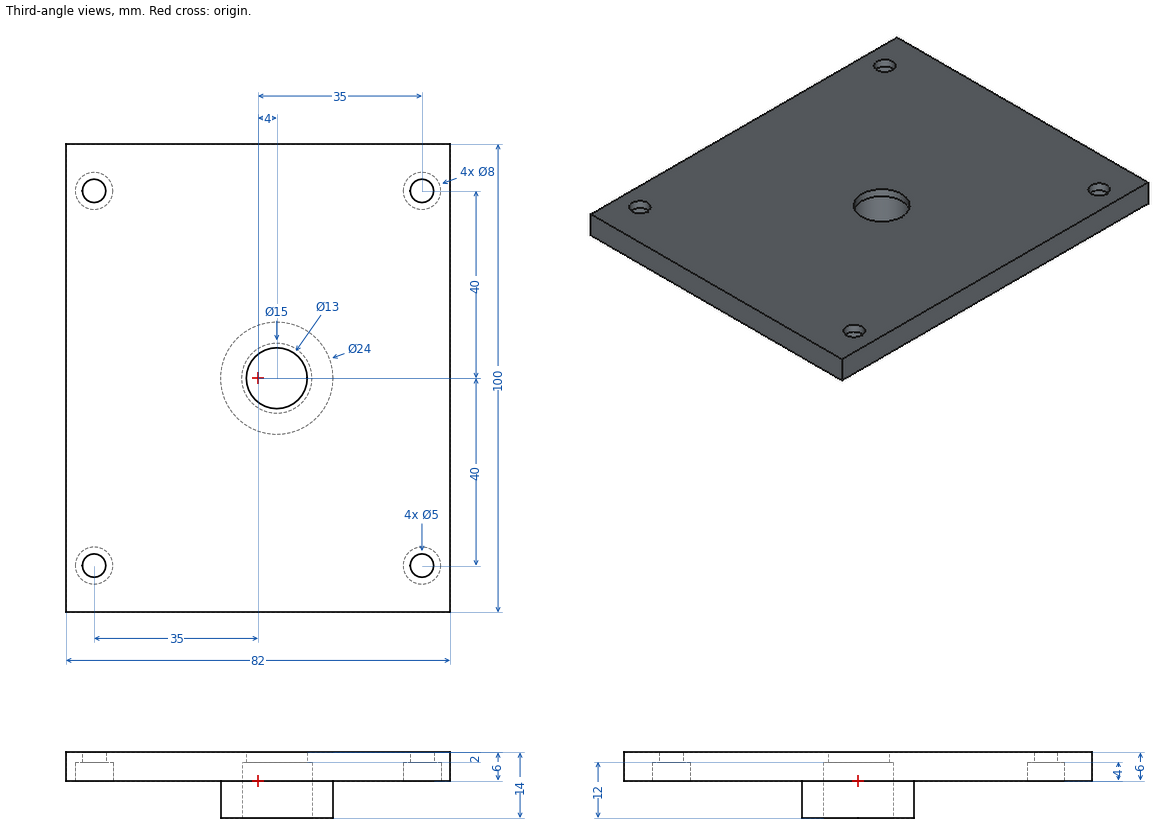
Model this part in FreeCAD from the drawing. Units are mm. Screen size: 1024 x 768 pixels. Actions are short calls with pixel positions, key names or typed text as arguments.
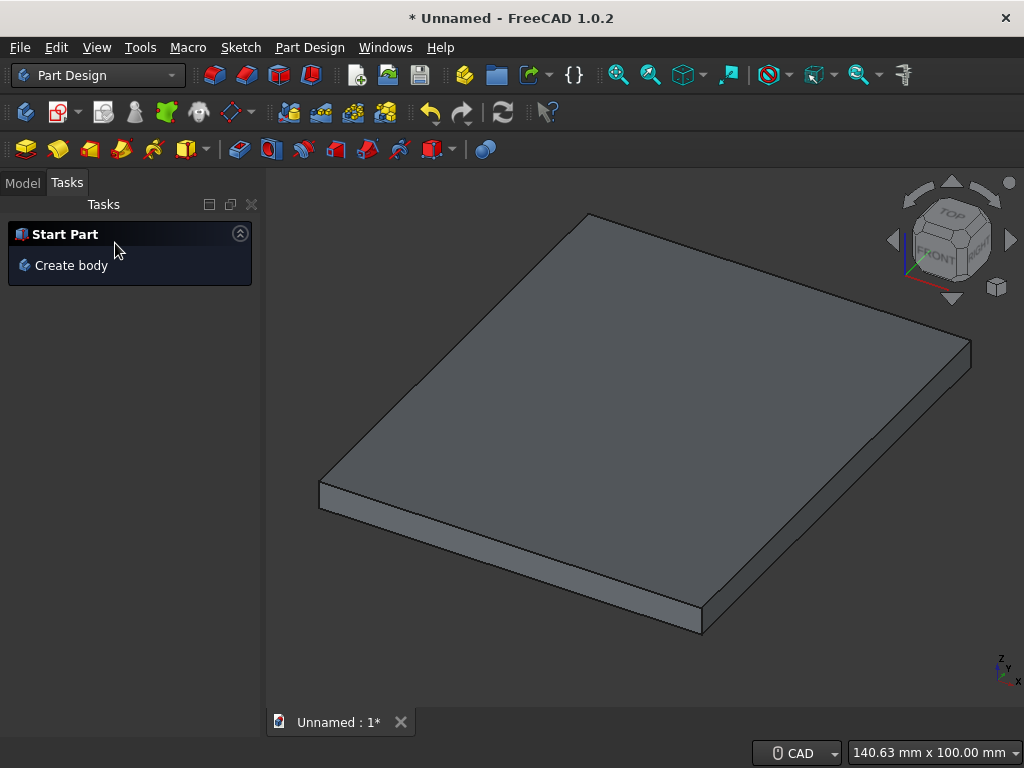
key(5)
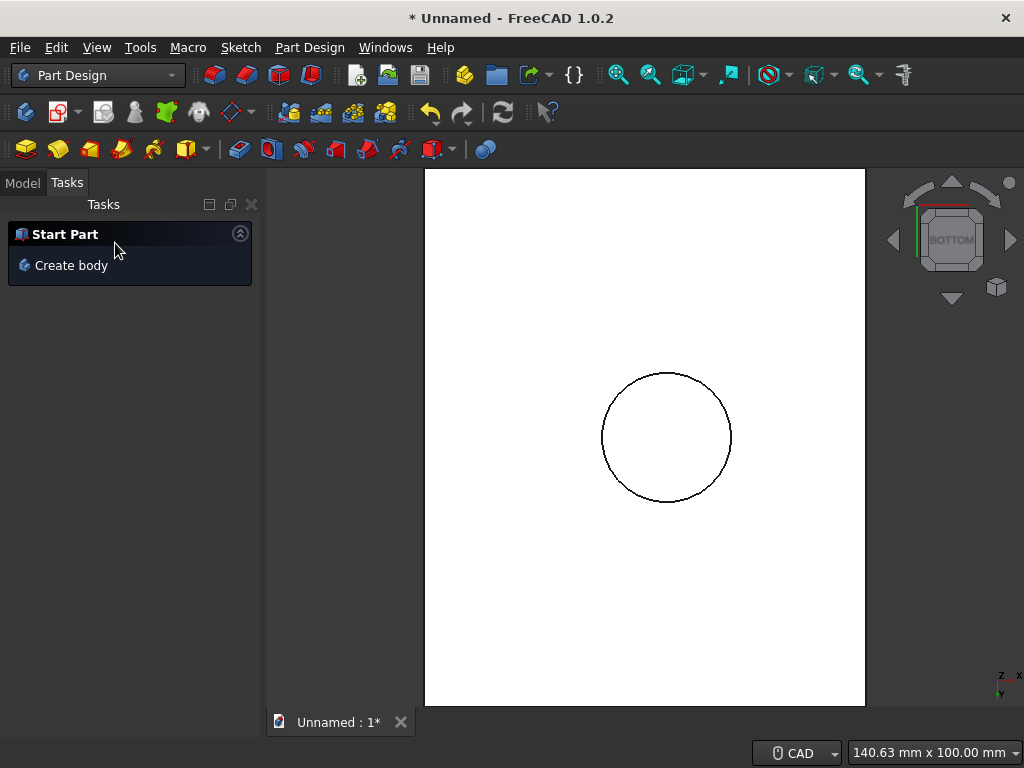
click(620, 76)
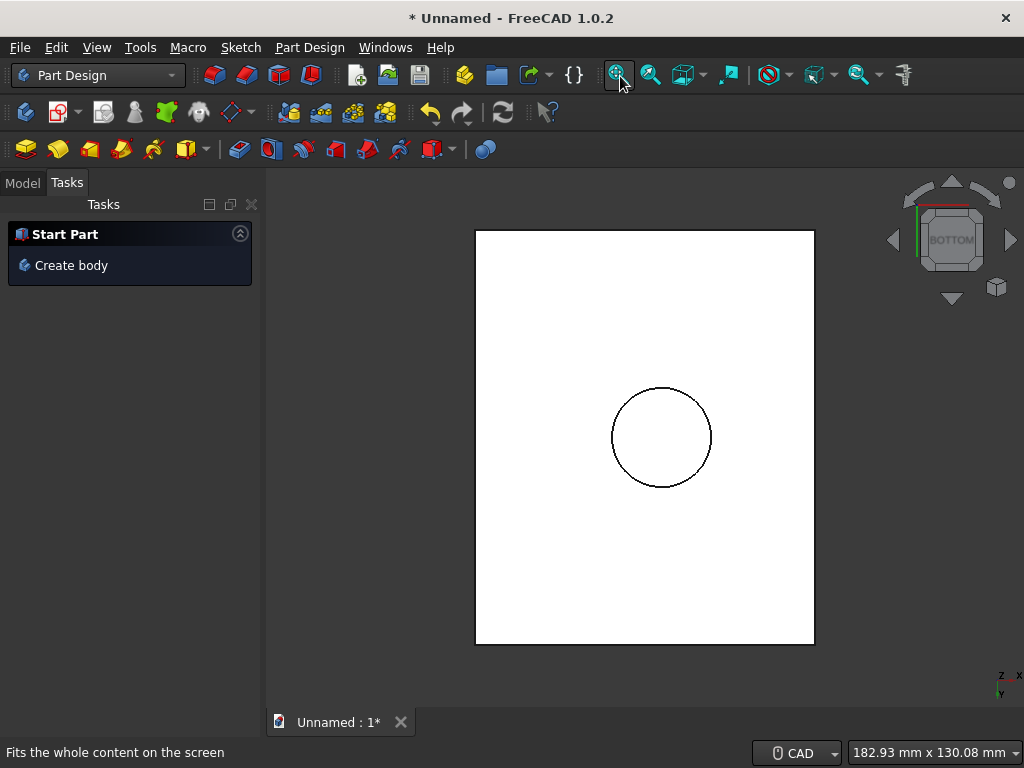
click(596, 555)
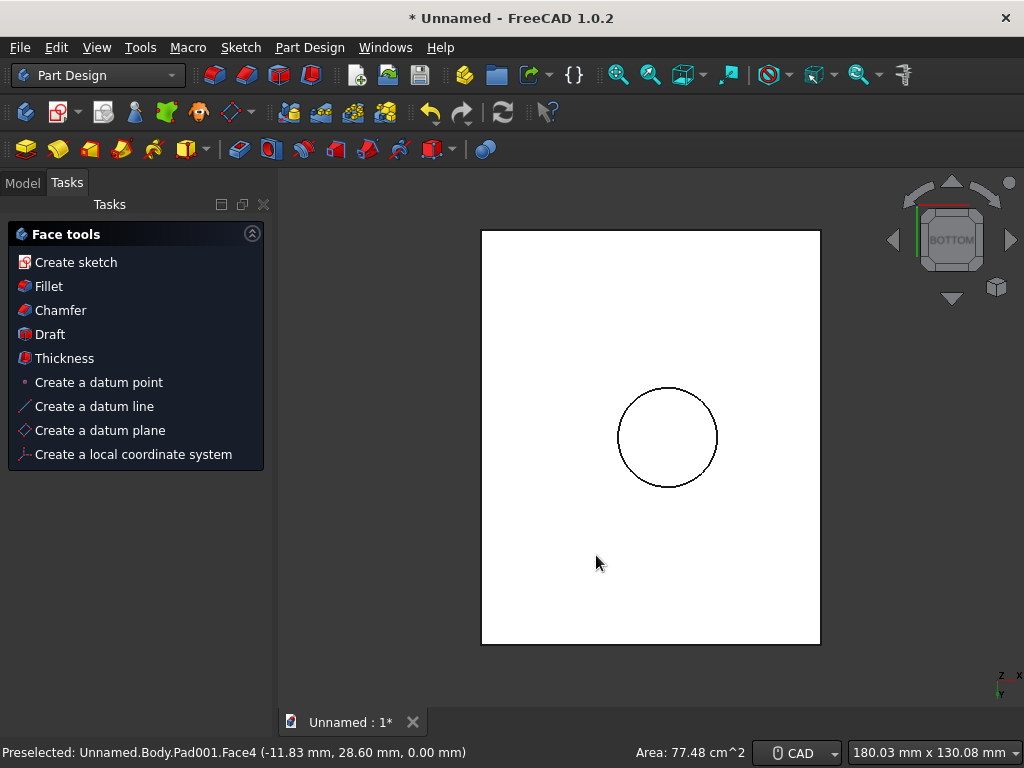
click(58, 112)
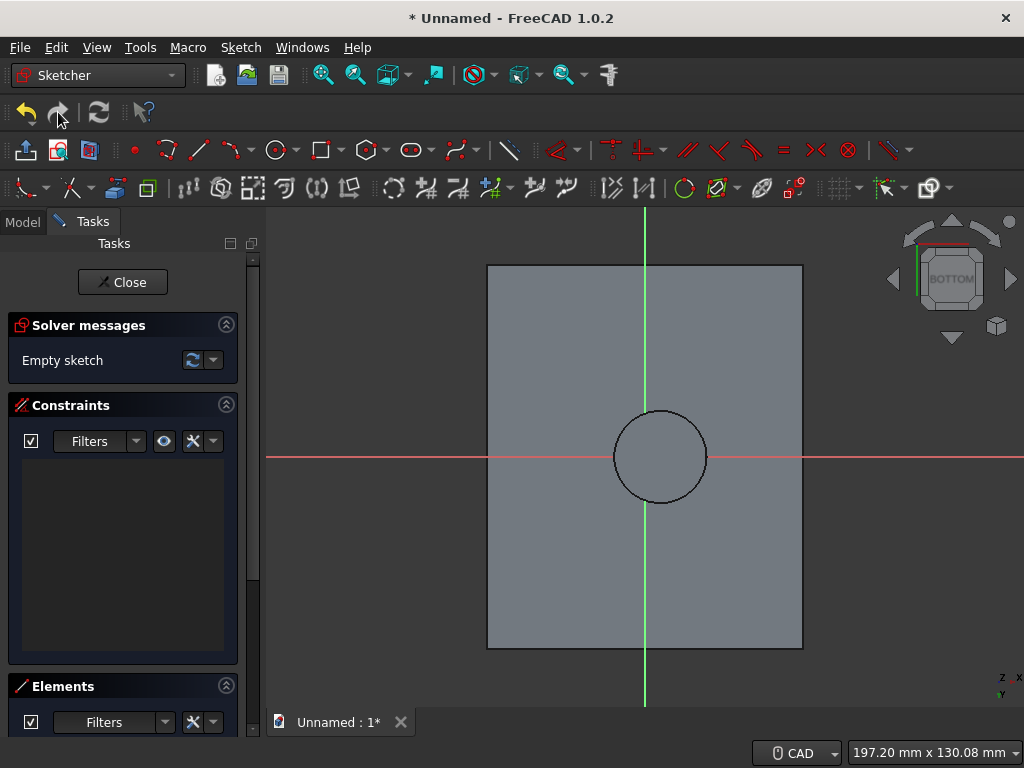
click(276, 150)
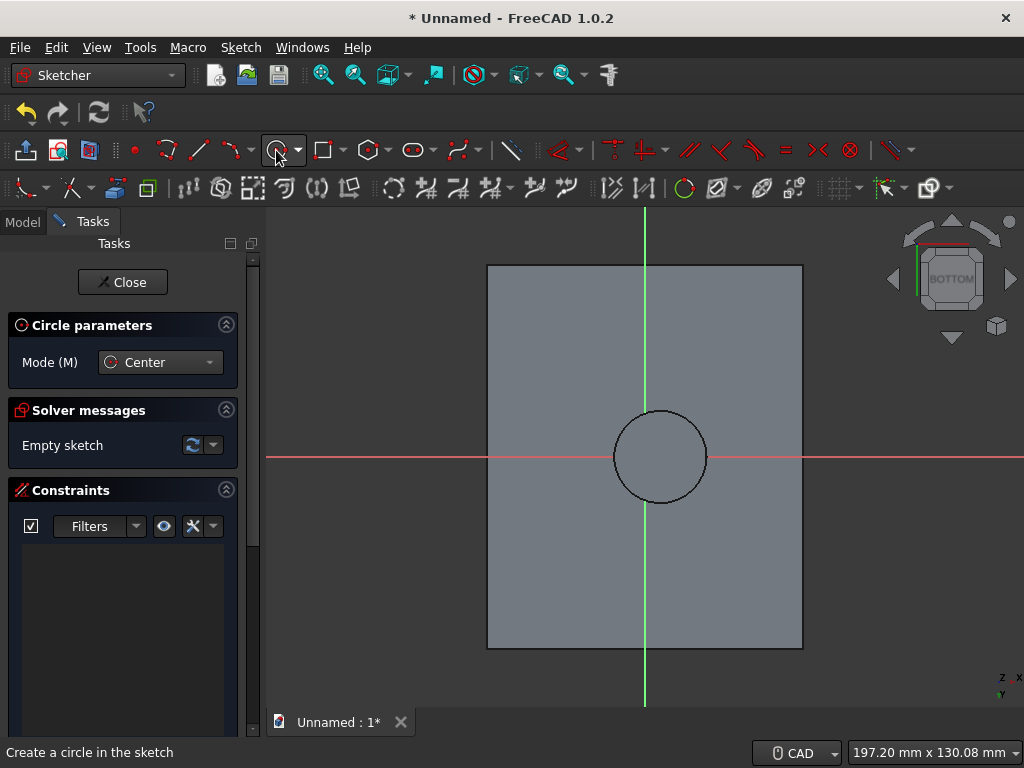
scroll(780, 611, up, 2)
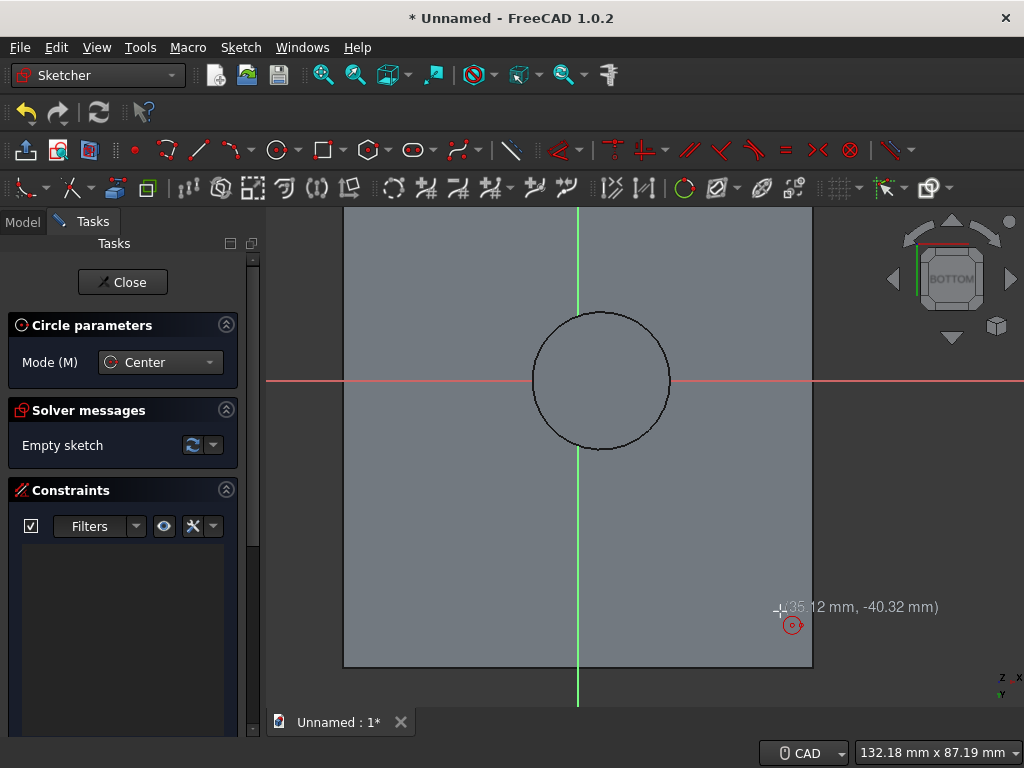
click(779, 610)
move(795, 594)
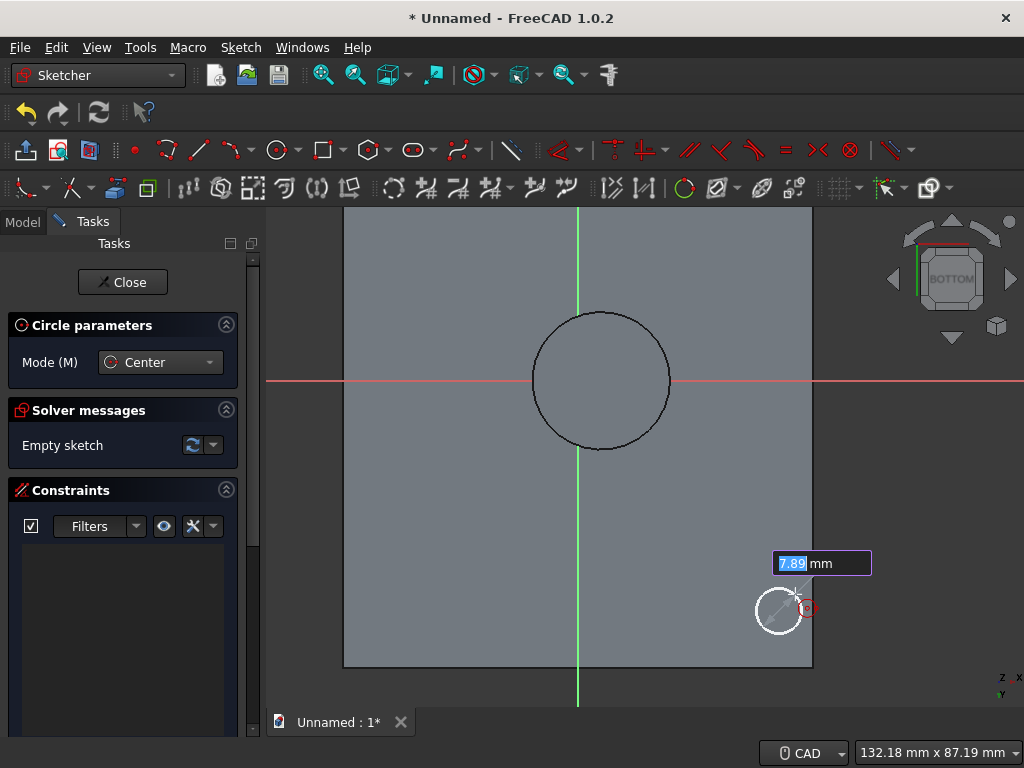
text(8)
key(Return)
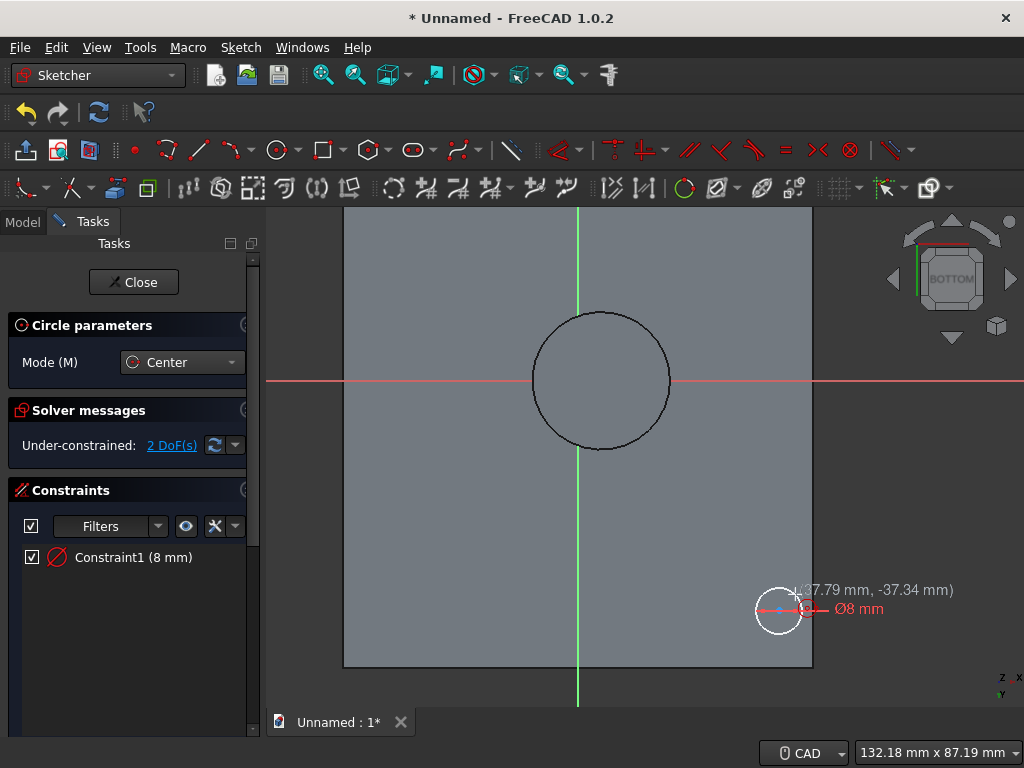
scroll(573, 612, down, 2)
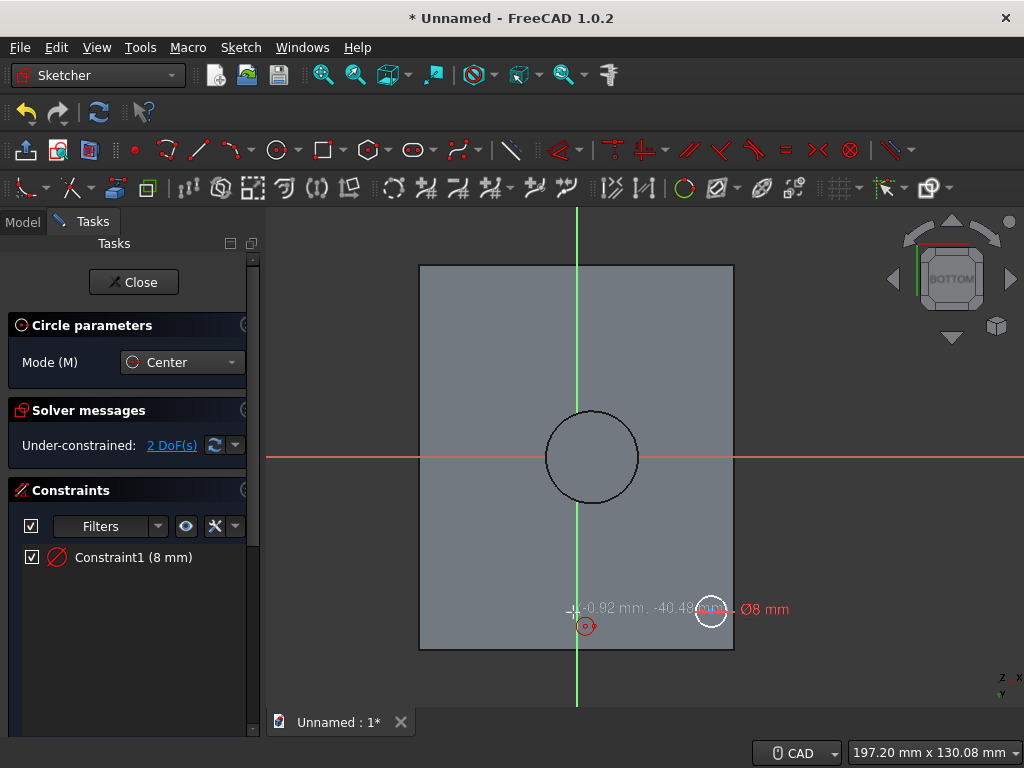
scroll(711, 304, up, 2)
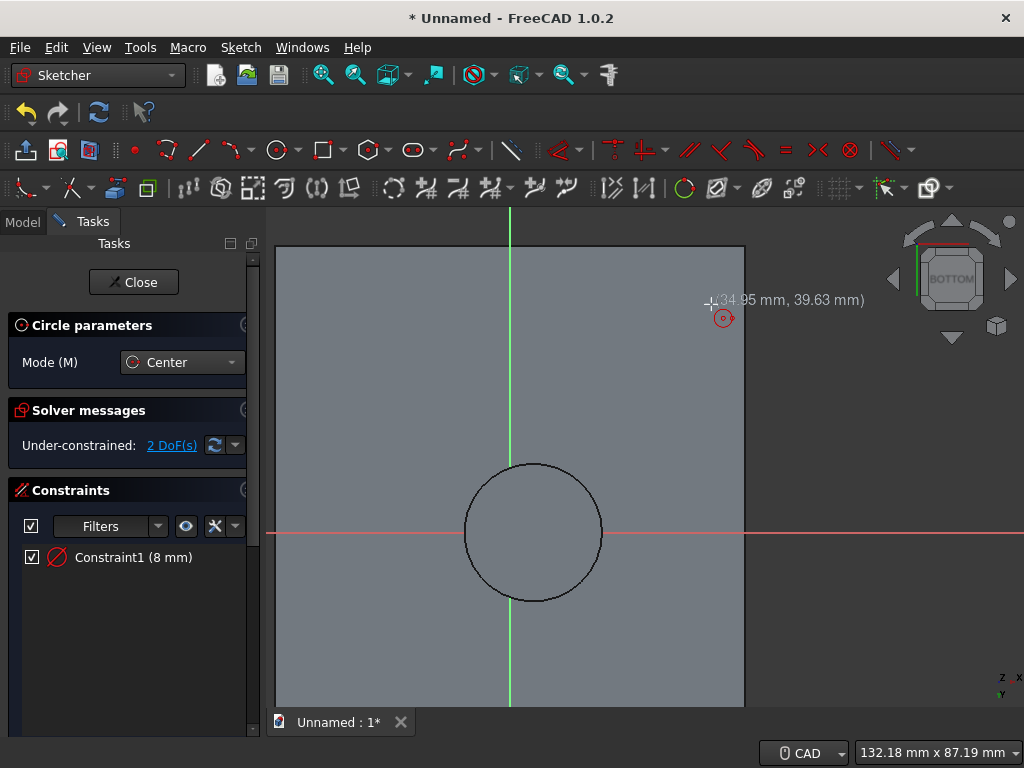
click(711, 303)
move(727, 287)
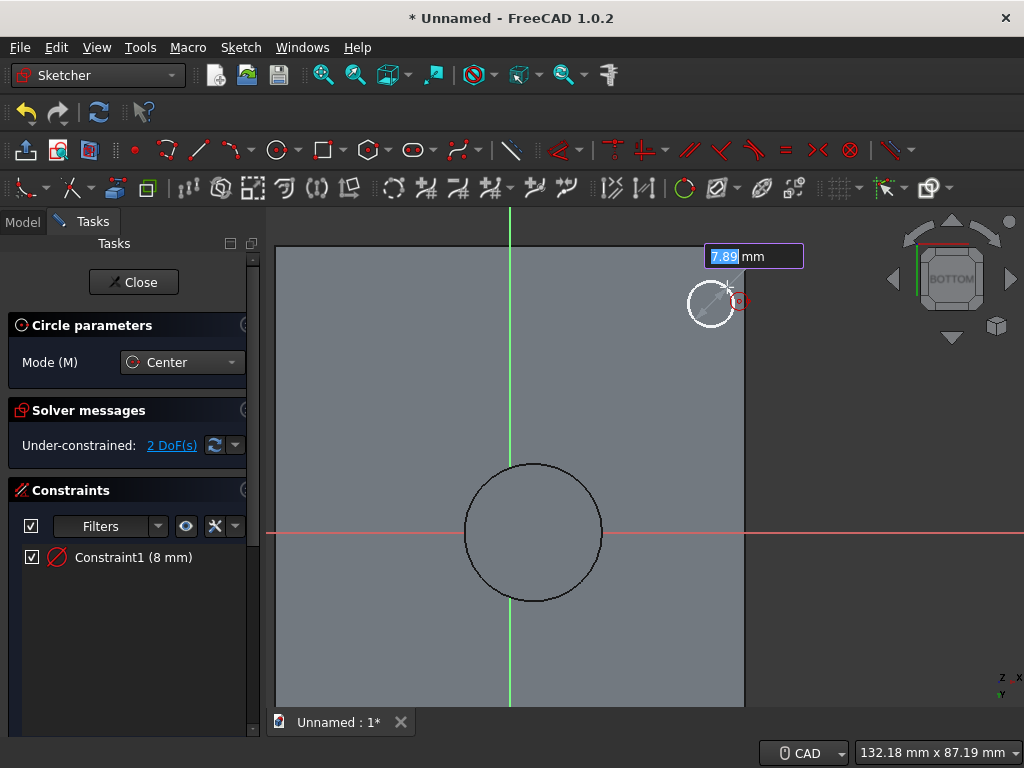
text(8)
key(Return)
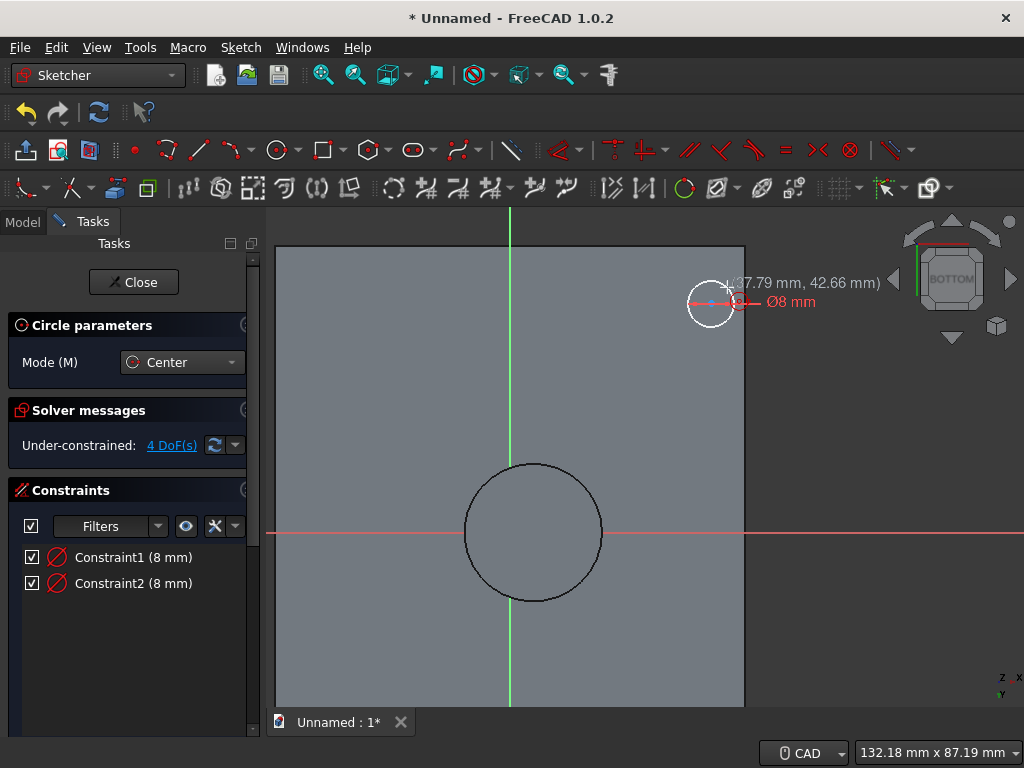
click(310, 303)
move(326, 287)